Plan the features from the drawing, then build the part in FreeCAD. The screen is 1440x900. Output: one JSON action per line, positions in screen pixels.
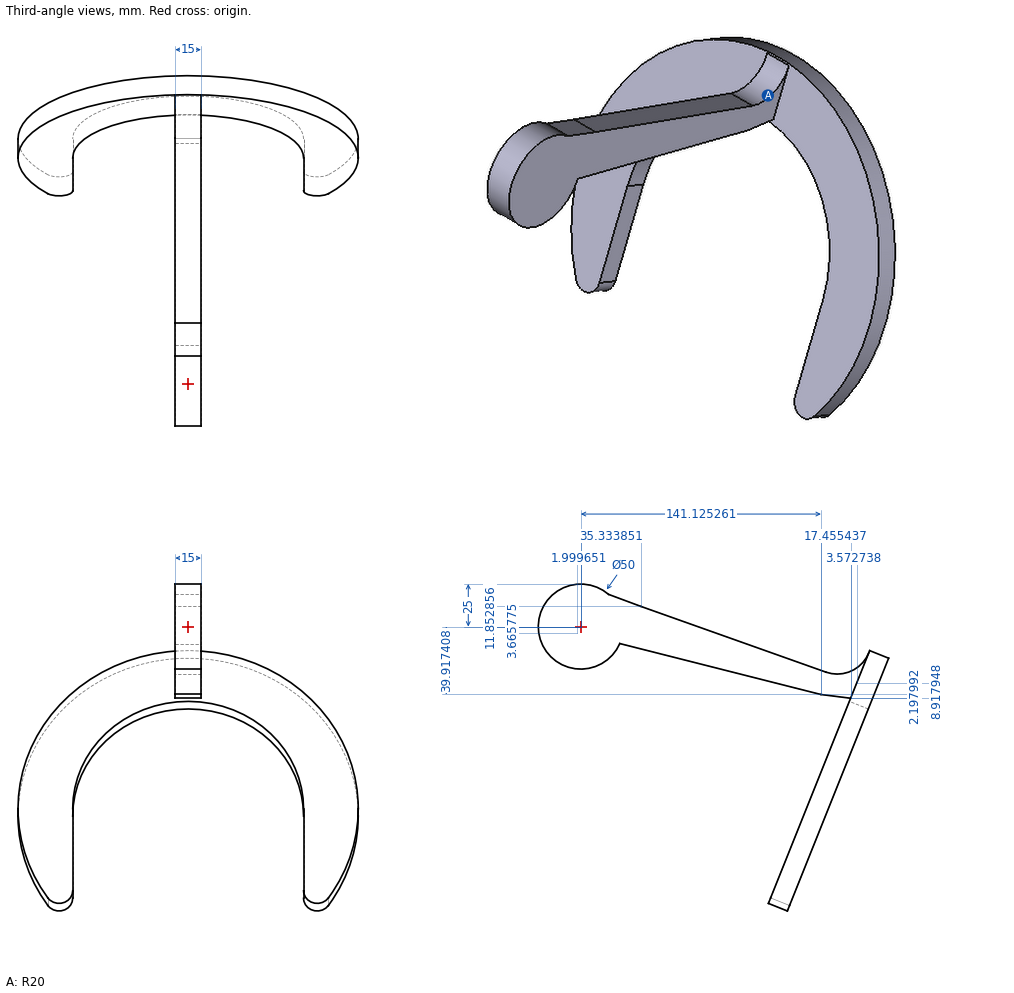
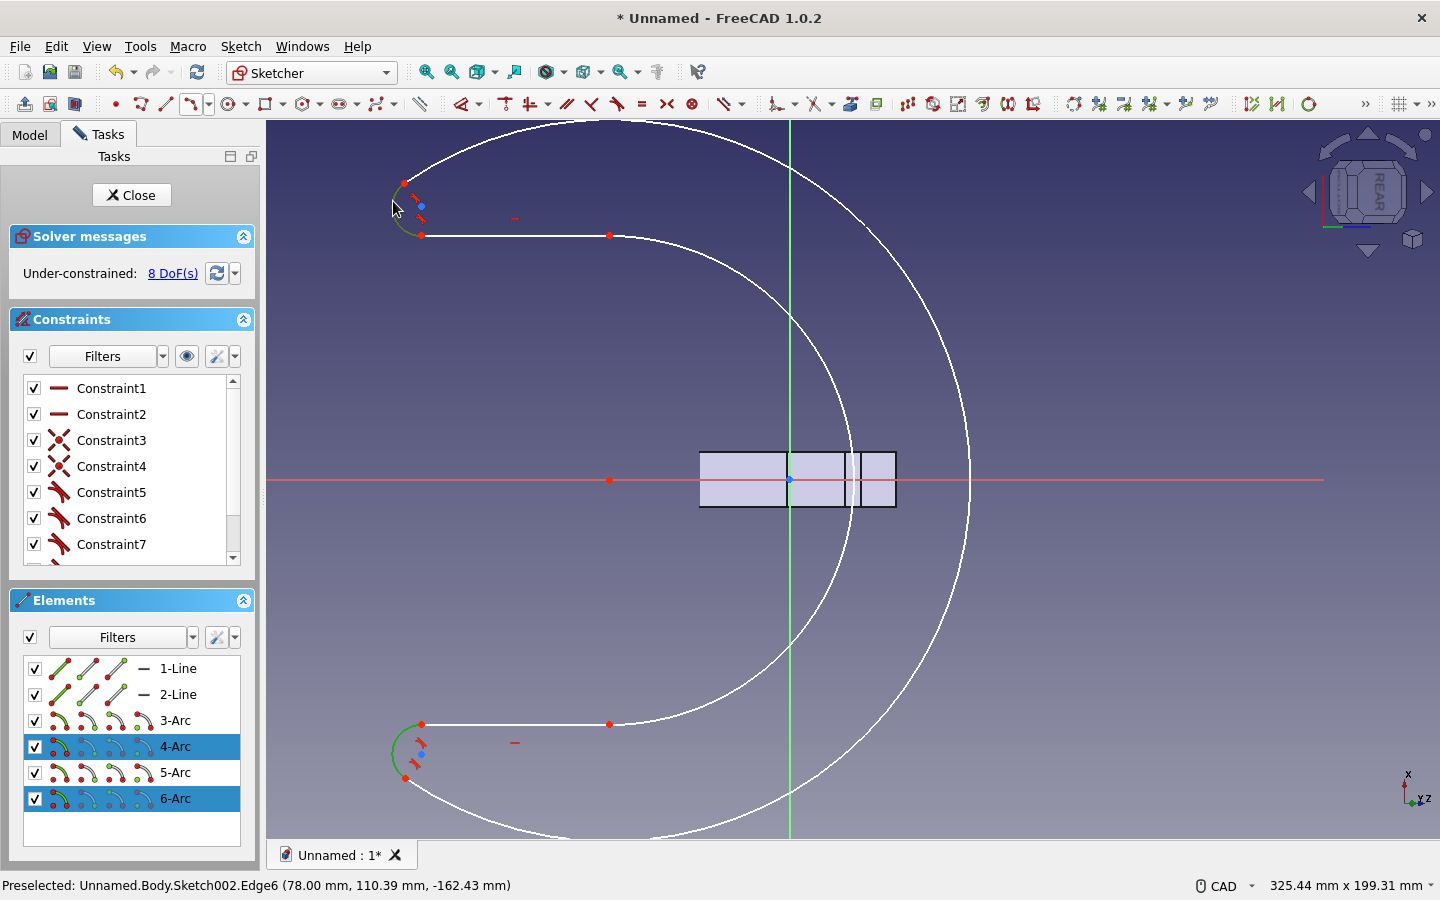
{"action": "key", "text": "e"}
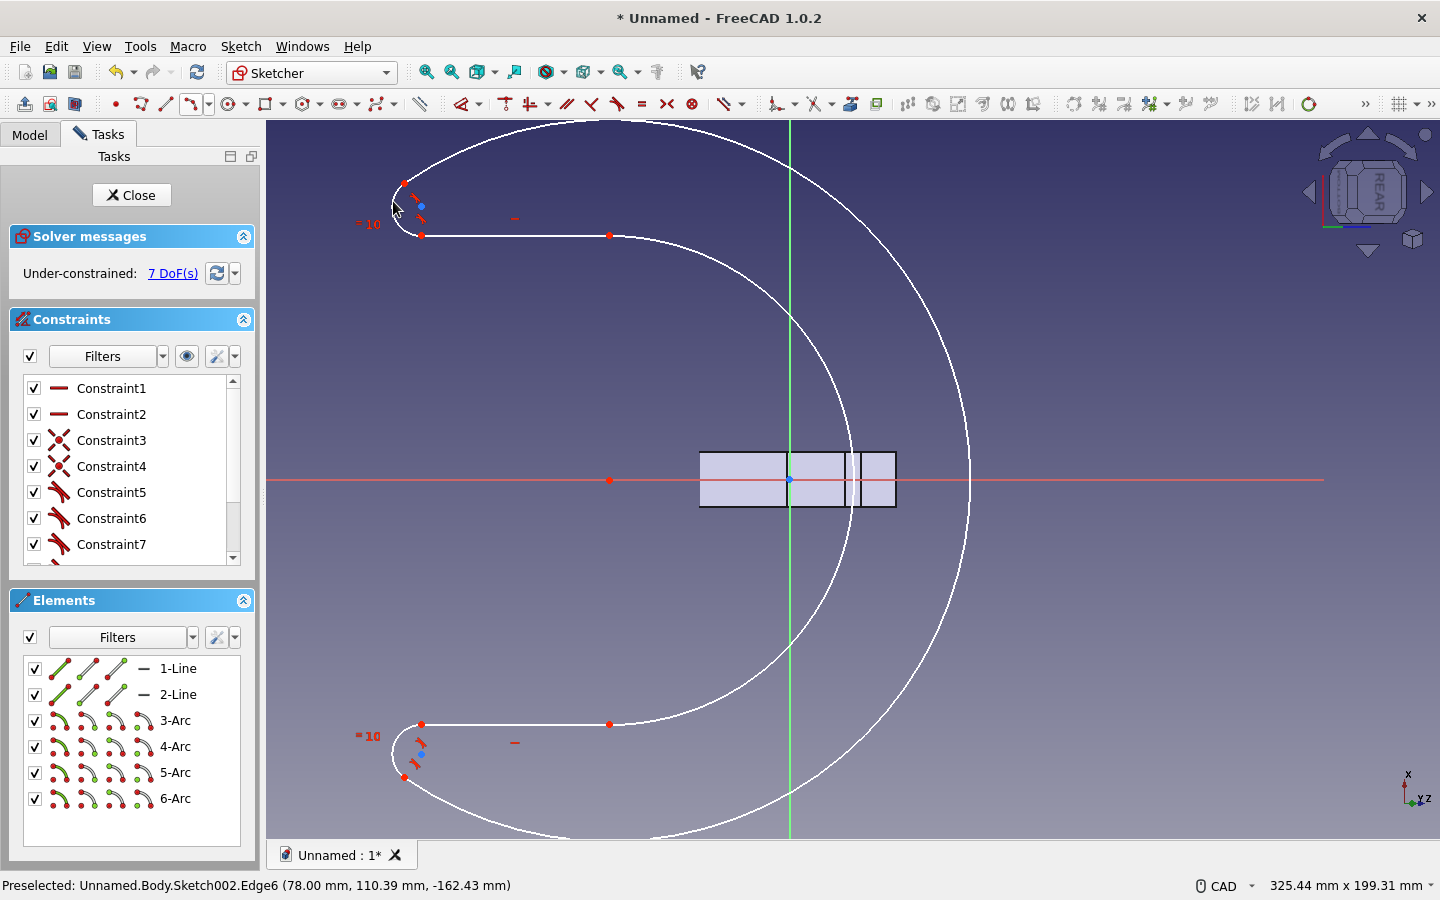
{"action": "left_click", "coordinate": [609, 480]}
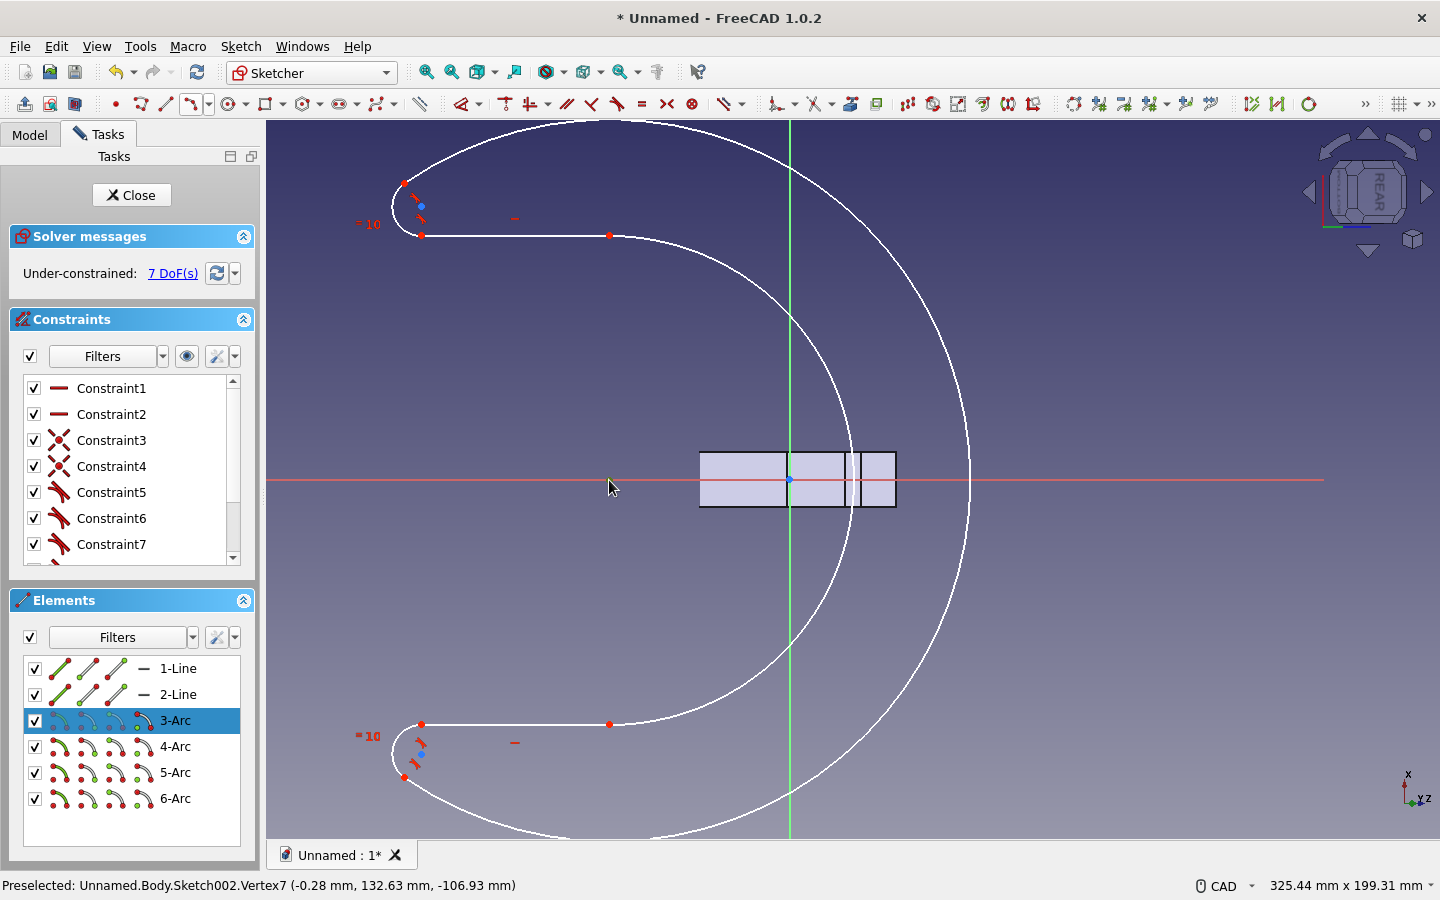
{"action": "left_click", "coordinate": [364, 479]}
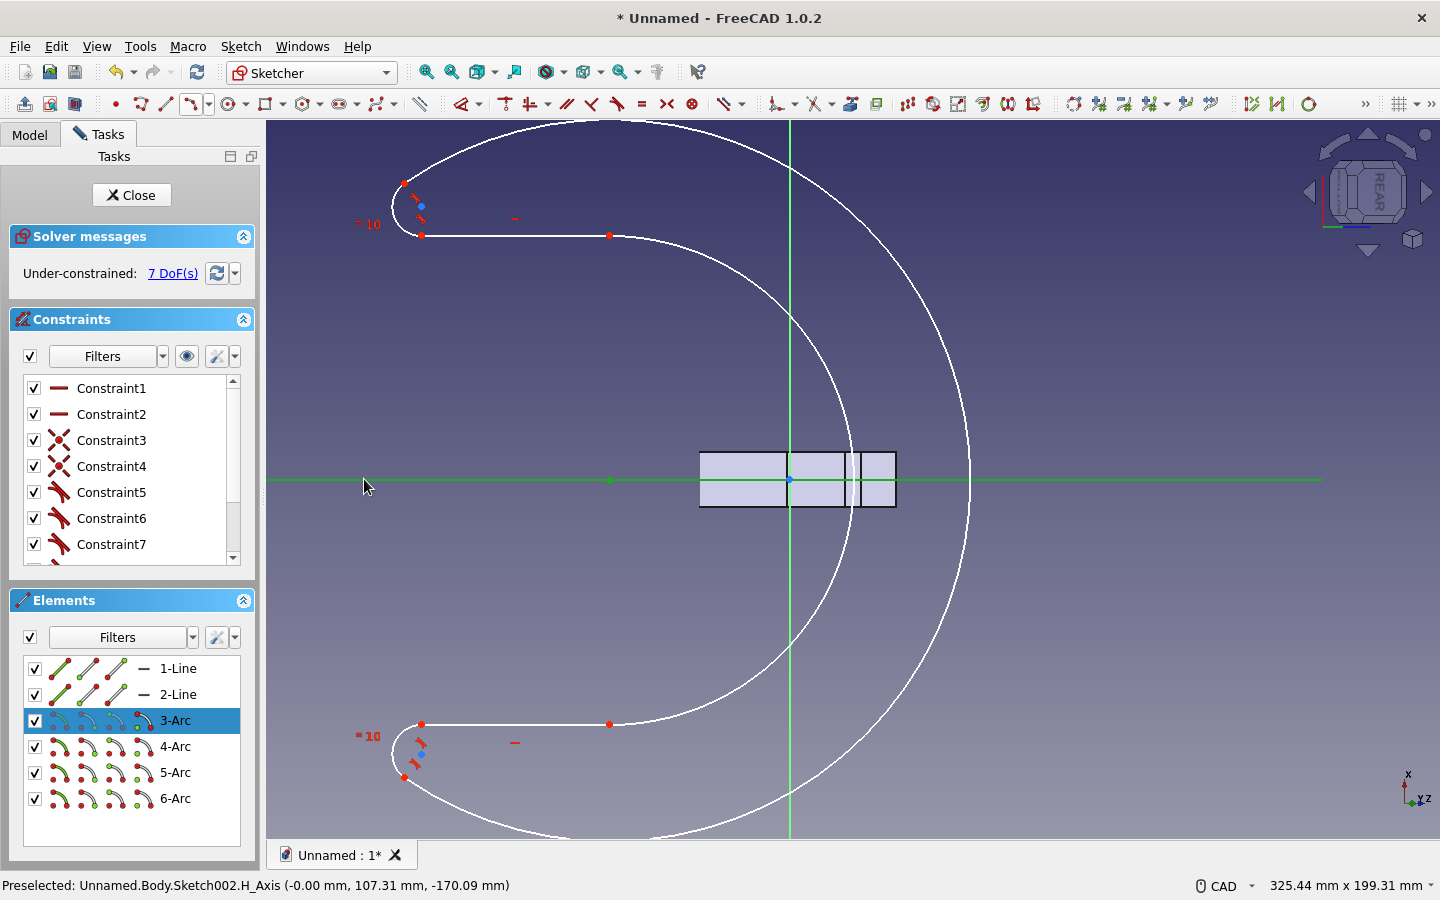
{"action": "key", "text": "c"}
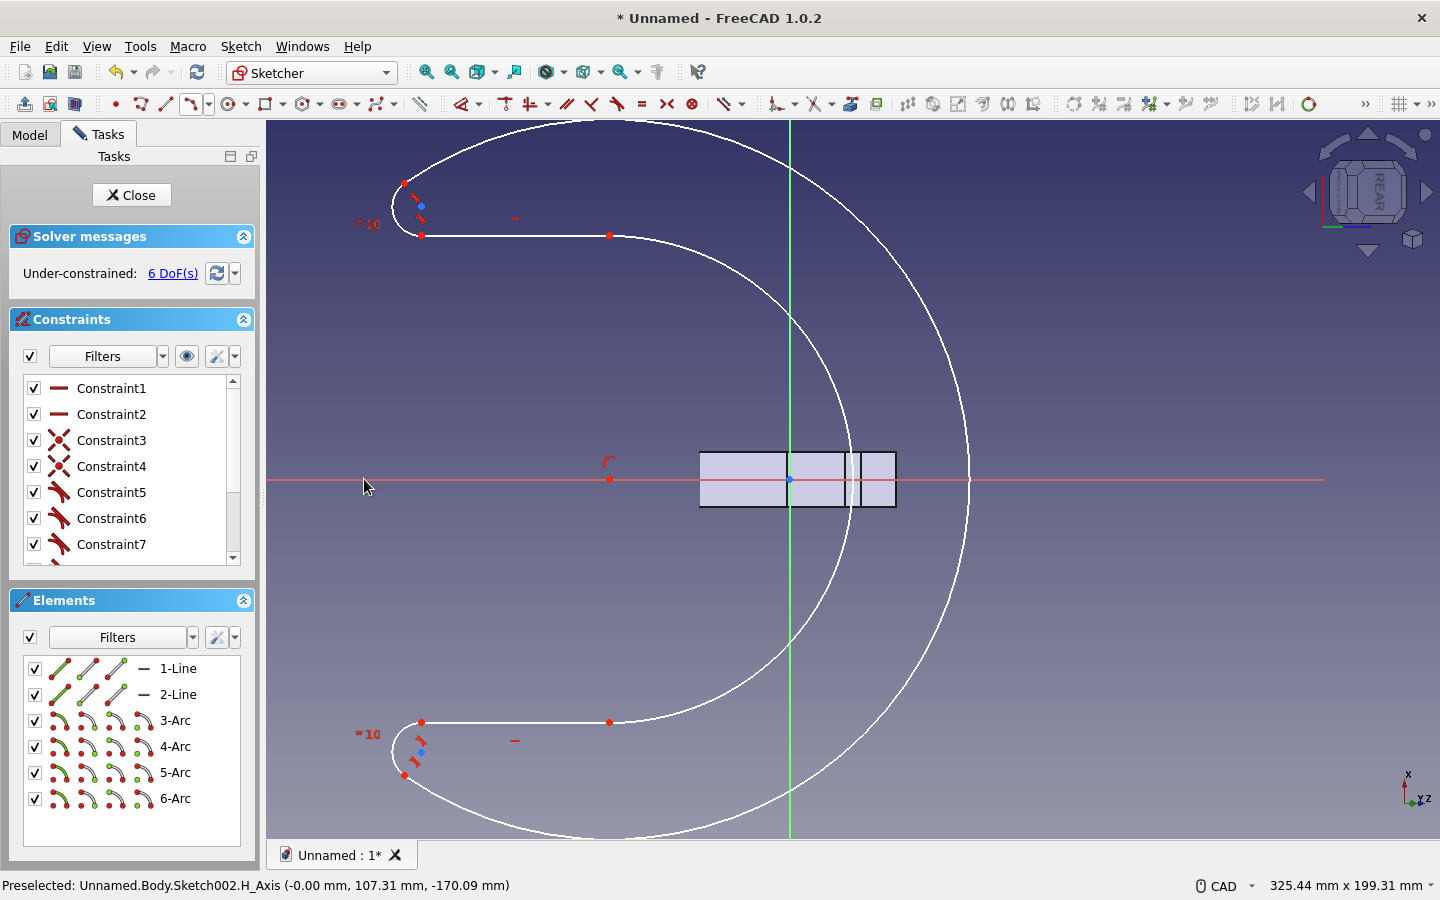
{"action": "left_click", "coordinate": [460, 104]}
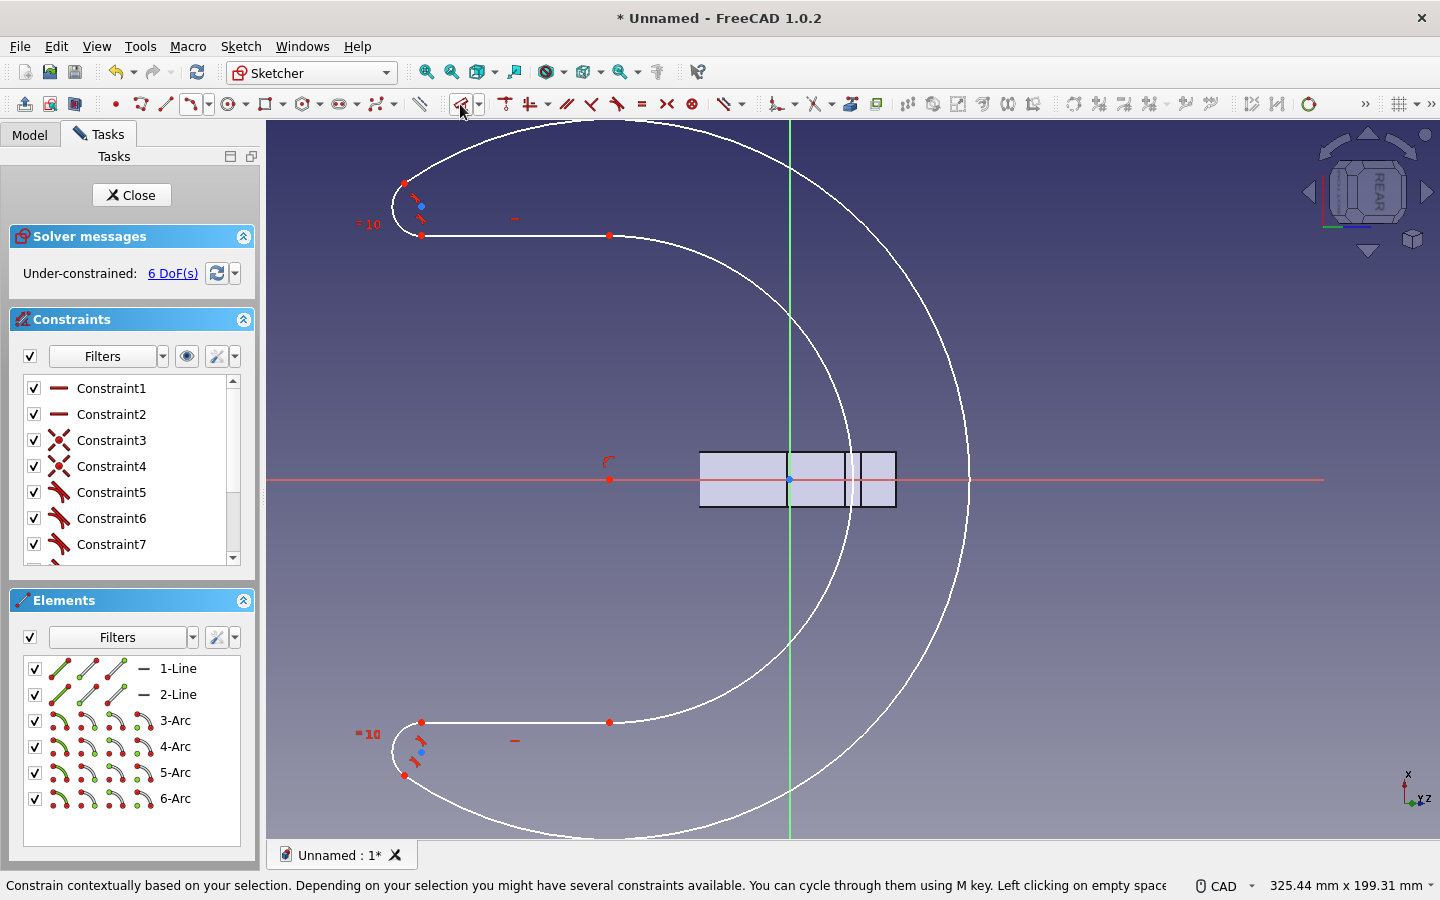
{"action": "left_click", "coordinate": [806, 623]}
{"action": "left_click", "coordinate": [832, 642]}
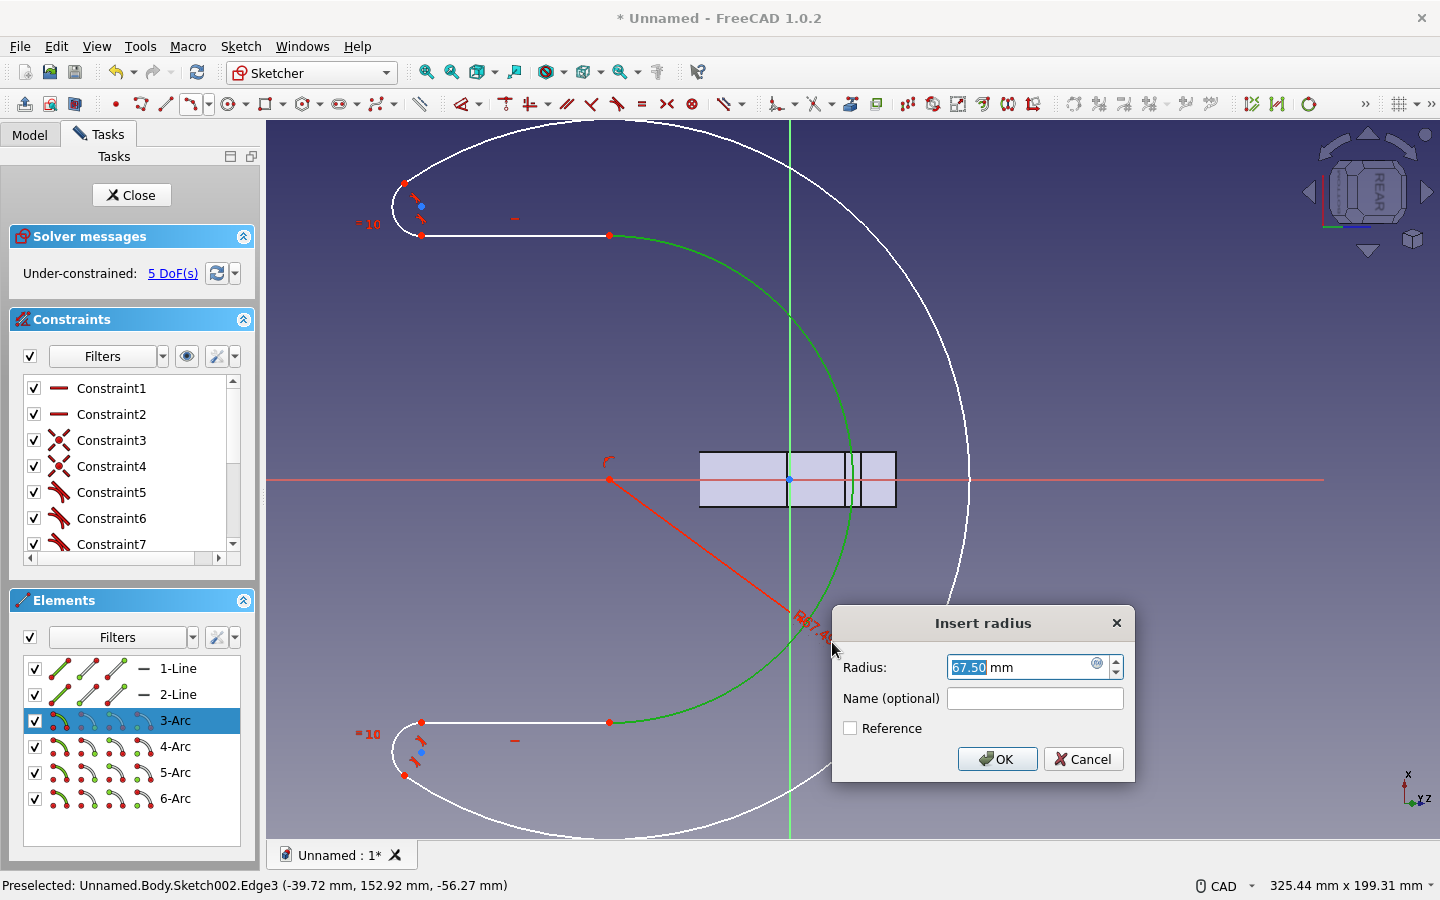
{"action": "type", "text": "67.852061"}
{"action": "key", "text": "Return"}